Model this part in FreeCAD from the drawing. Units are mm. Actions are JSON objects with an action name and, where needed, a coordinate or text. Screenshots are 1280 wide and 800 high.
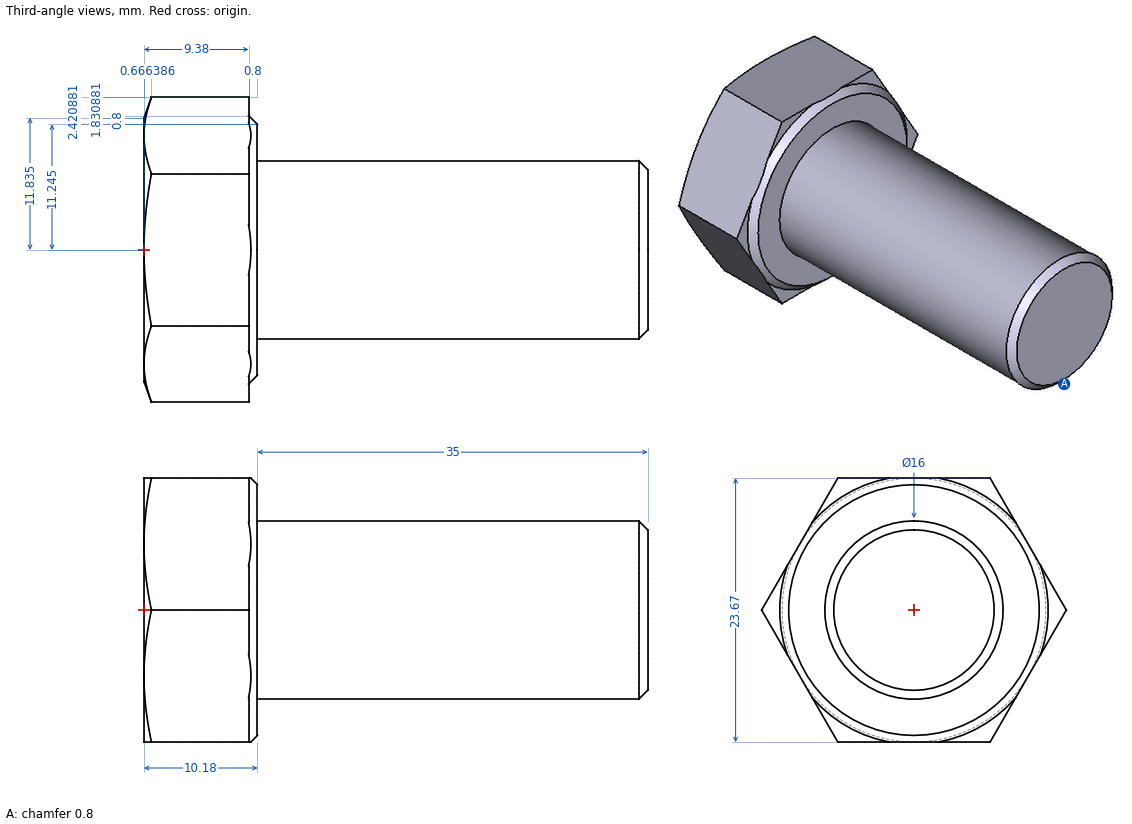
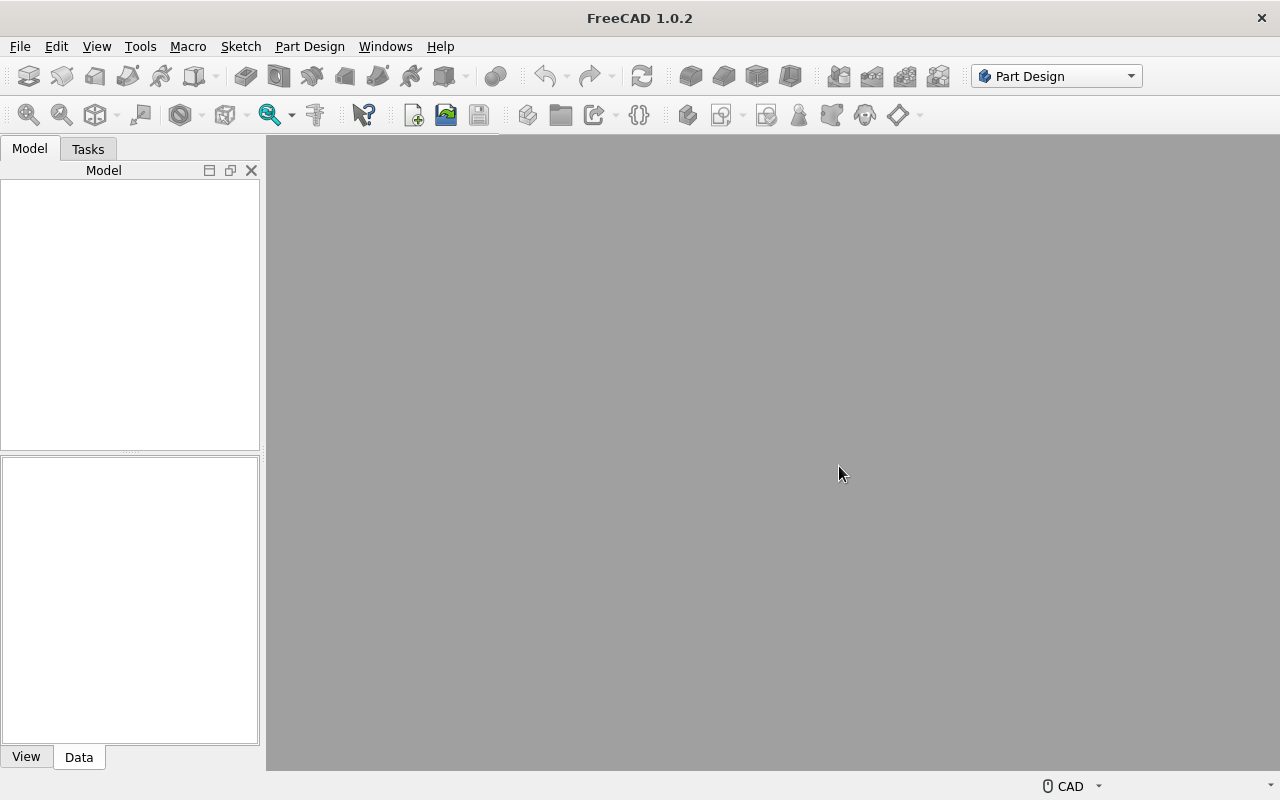
{"action": "key", "text": "ctrl+n"}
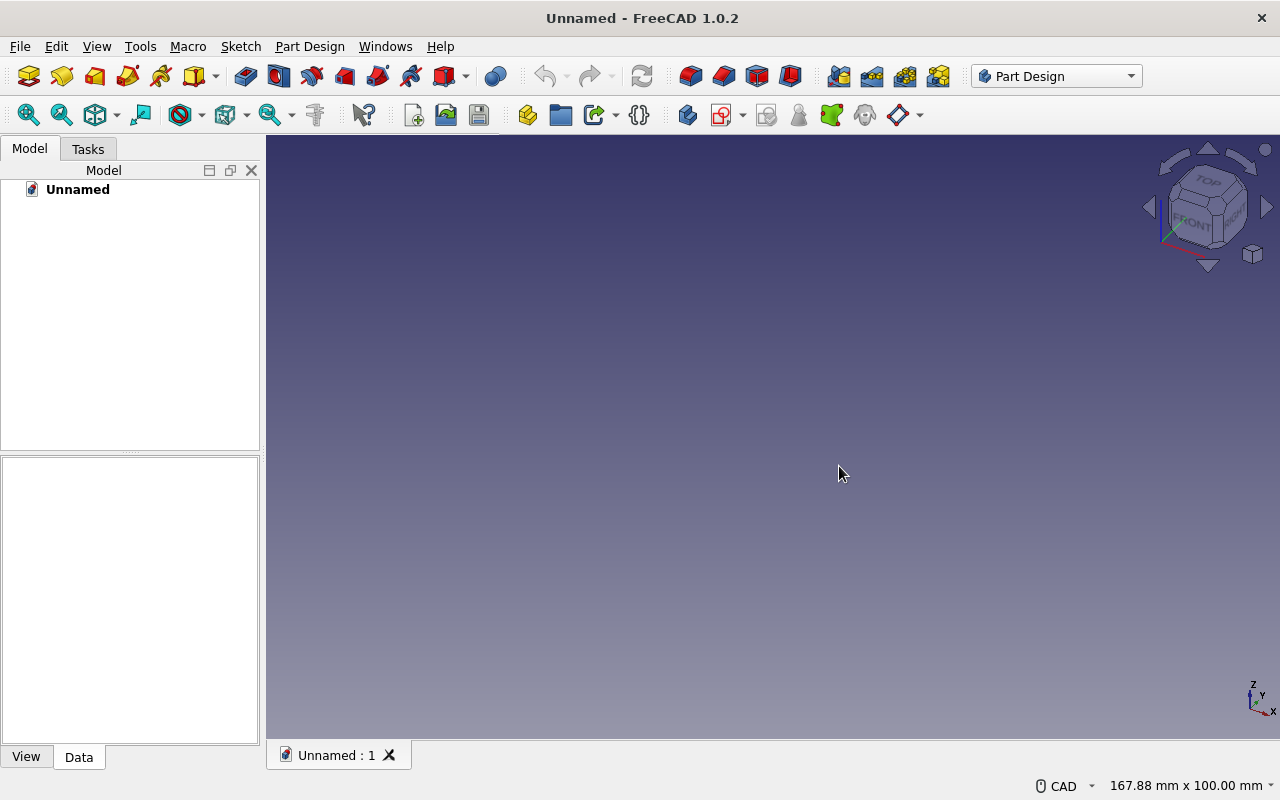
{"action": "left_click", "coordinate": [720, 116]}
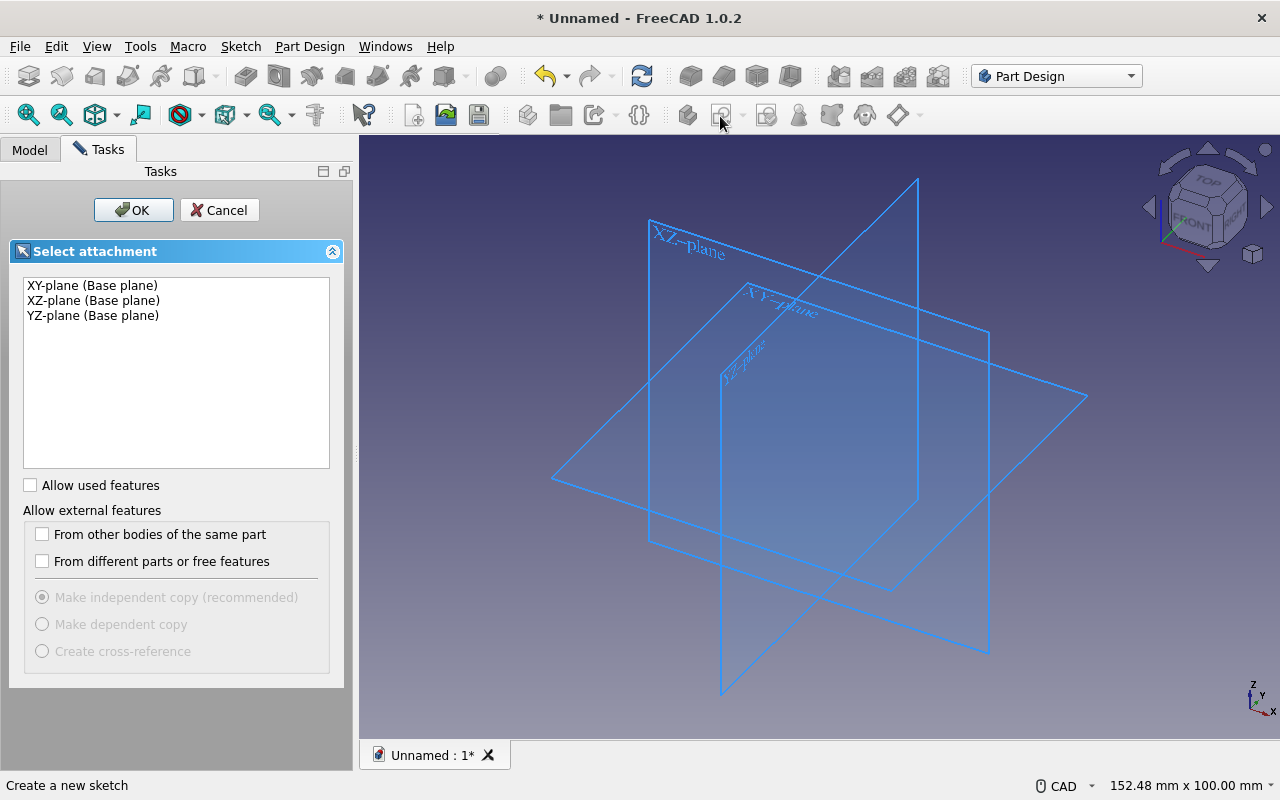
{"action": "left_click", "coordinate": [84, 316]}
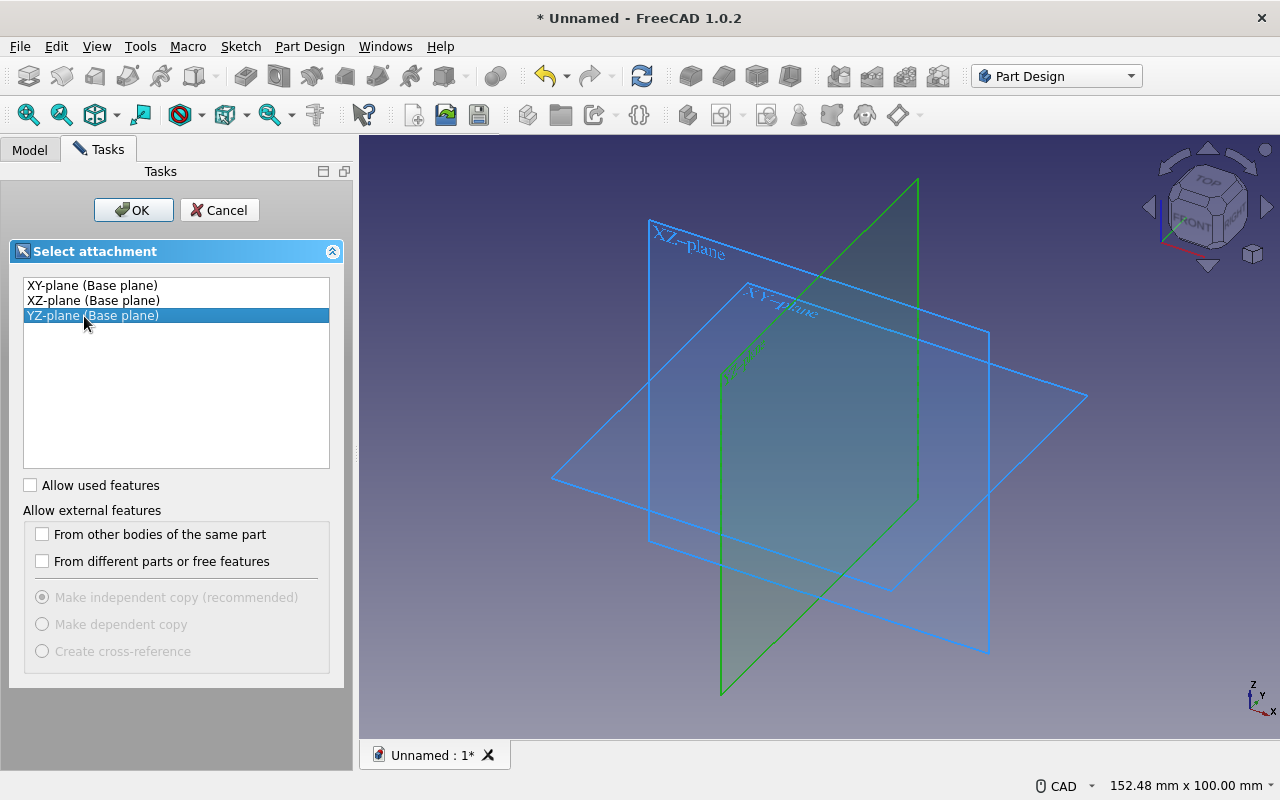
{"action": "left_click", "coordinate": [134, 210]}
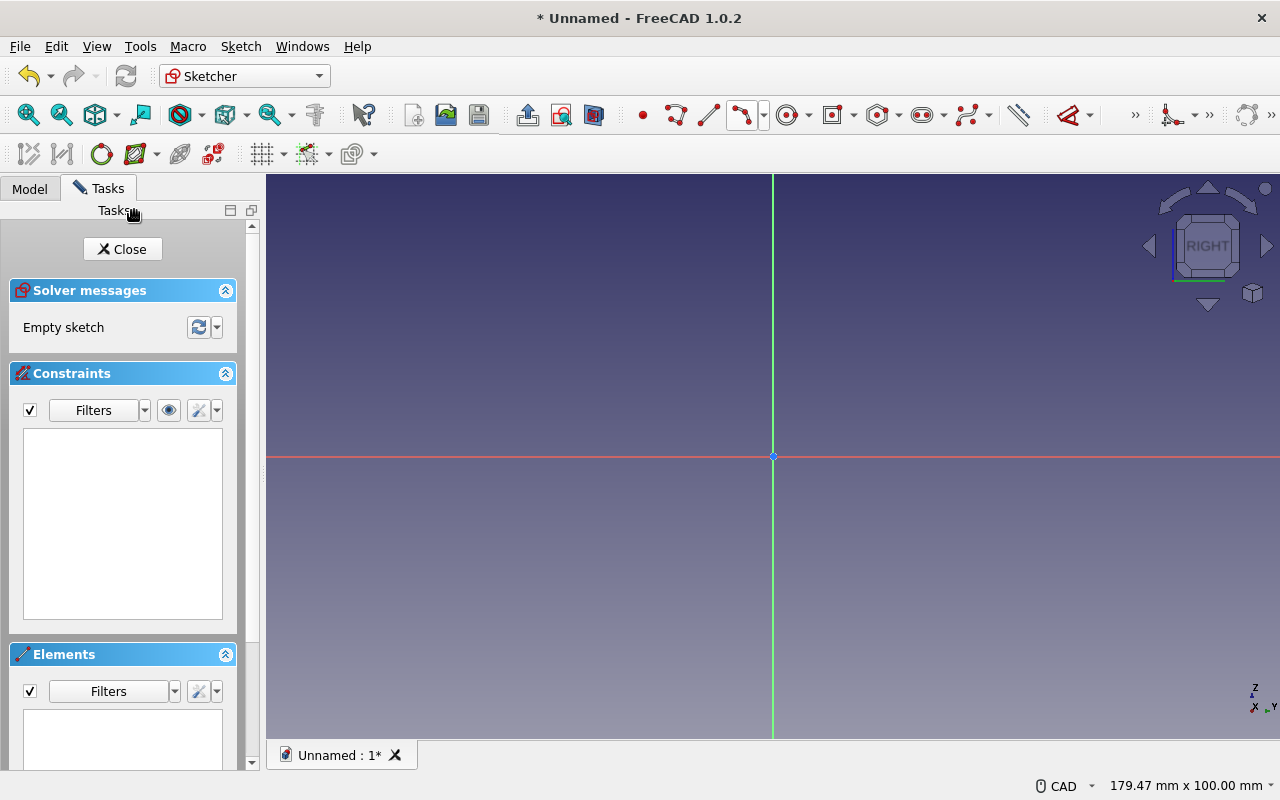
{"action": "scroll", "coordinate": [813, 456], "scroll_direction": "up", "scroll_amount": 5}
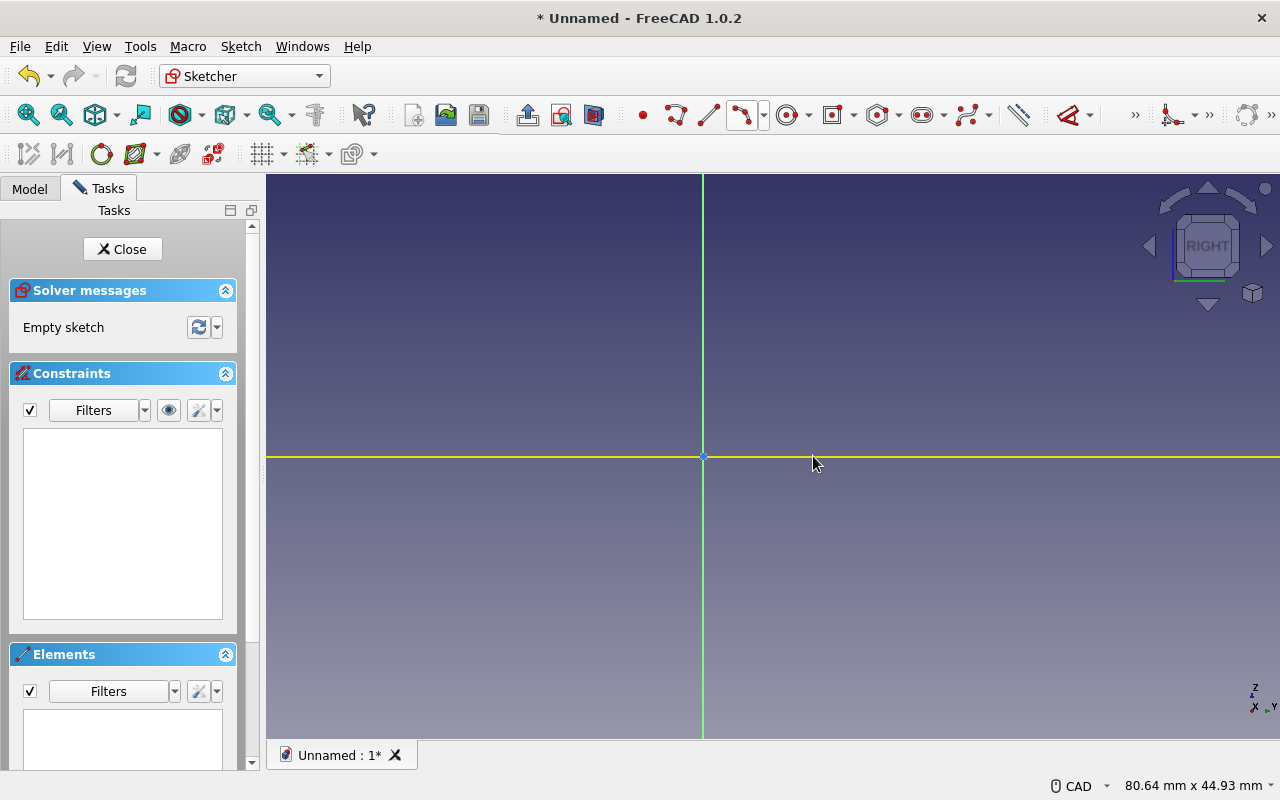
{"action": "left_click", "coordinate": [876, 116]}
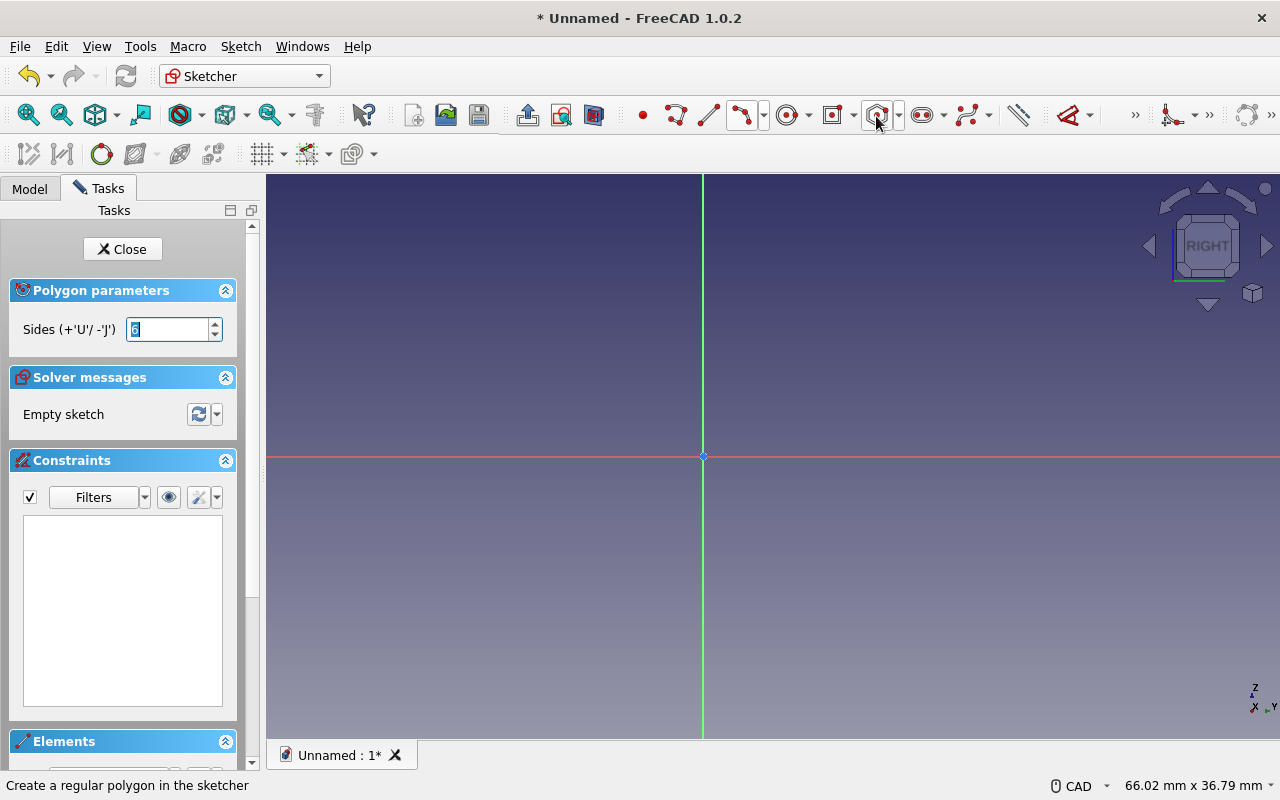
{"action": "left_click", "coordinate": [703, 456]}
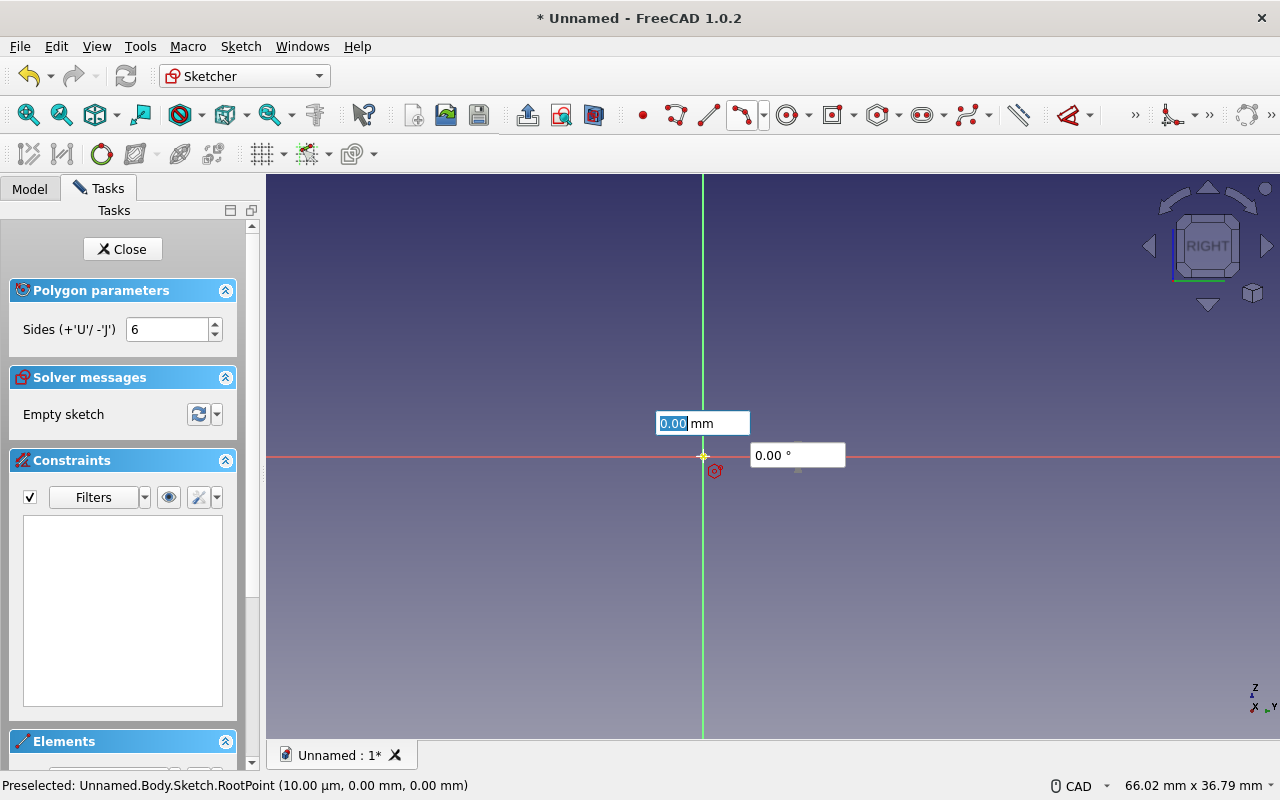
{"action": "left_click", "coordinate": [913, 456]}
{"action": "key", "text": "Escape"}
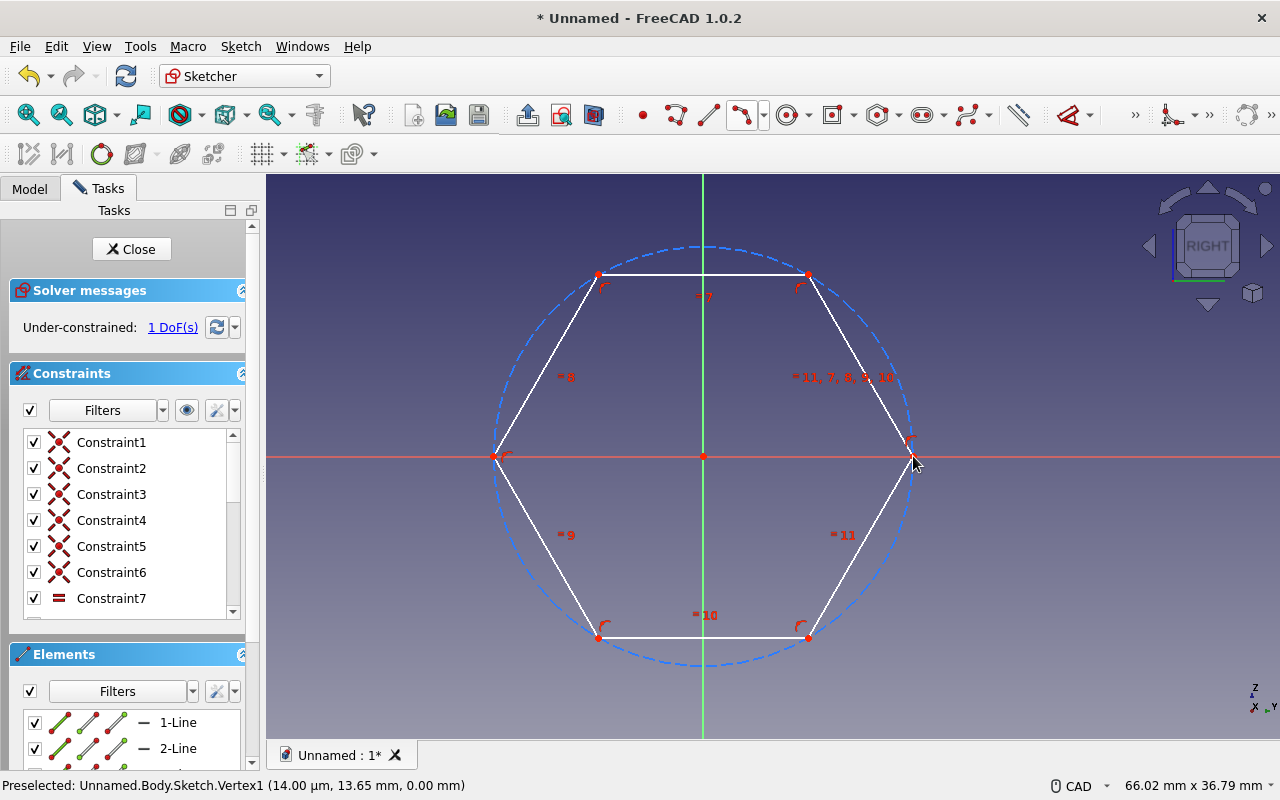
{"action": "key", "text": "d"}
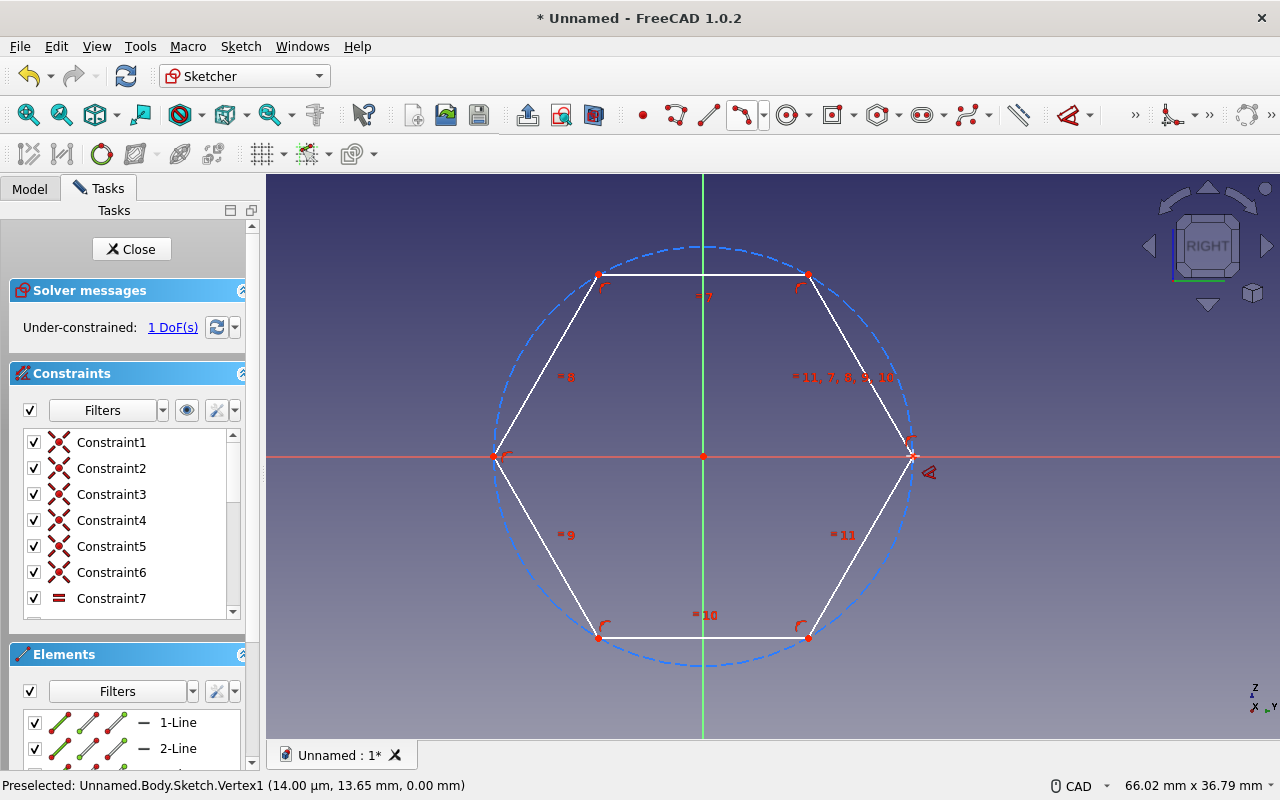
{"action": "left_click", "coordinate": [599, 638]}